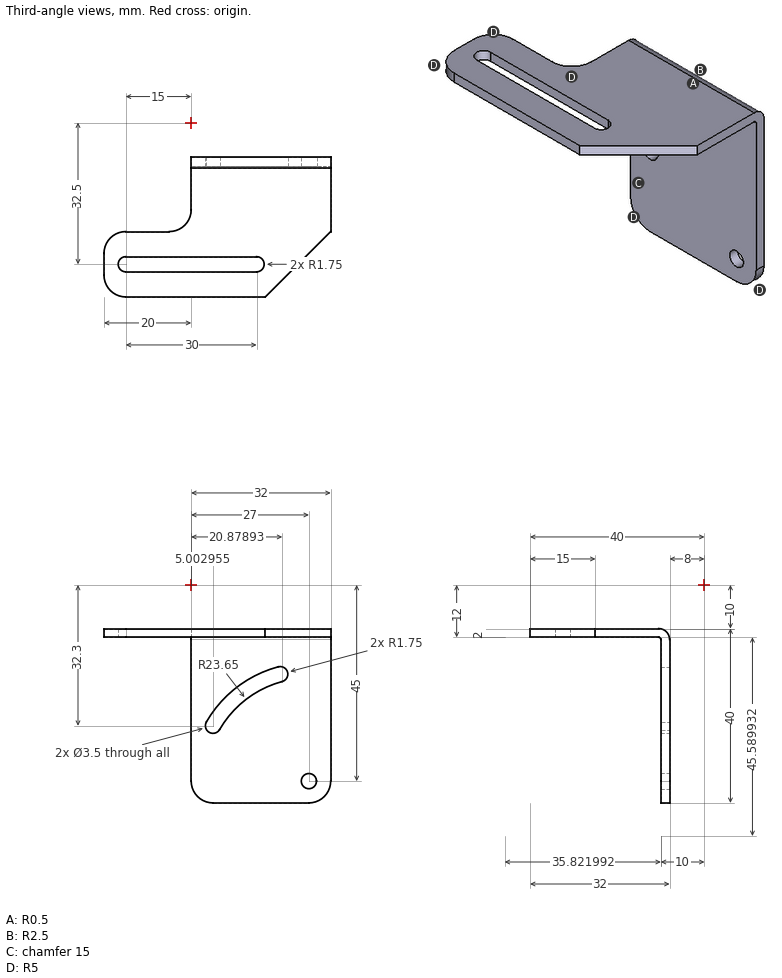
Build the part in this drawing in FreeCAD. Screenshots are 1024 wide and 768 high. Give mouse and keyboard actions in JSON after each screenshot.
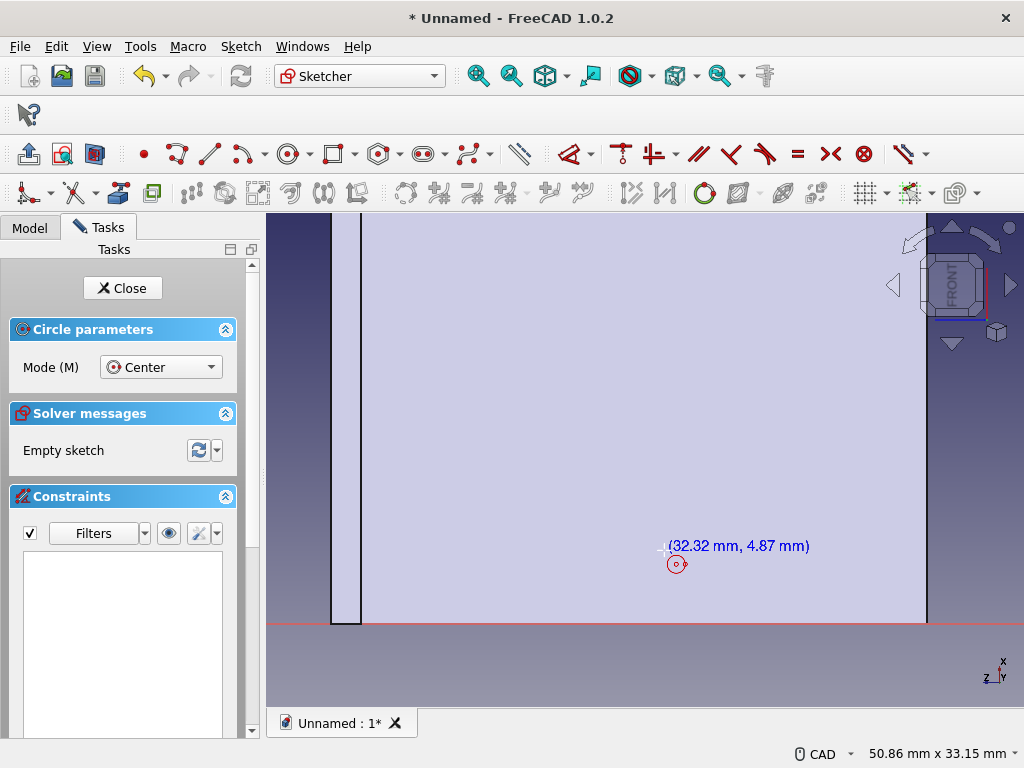
{"action": "left_click", "coordinate": [663, 549]}
{"action": "mouse_move", "coordinate": [682, 531]}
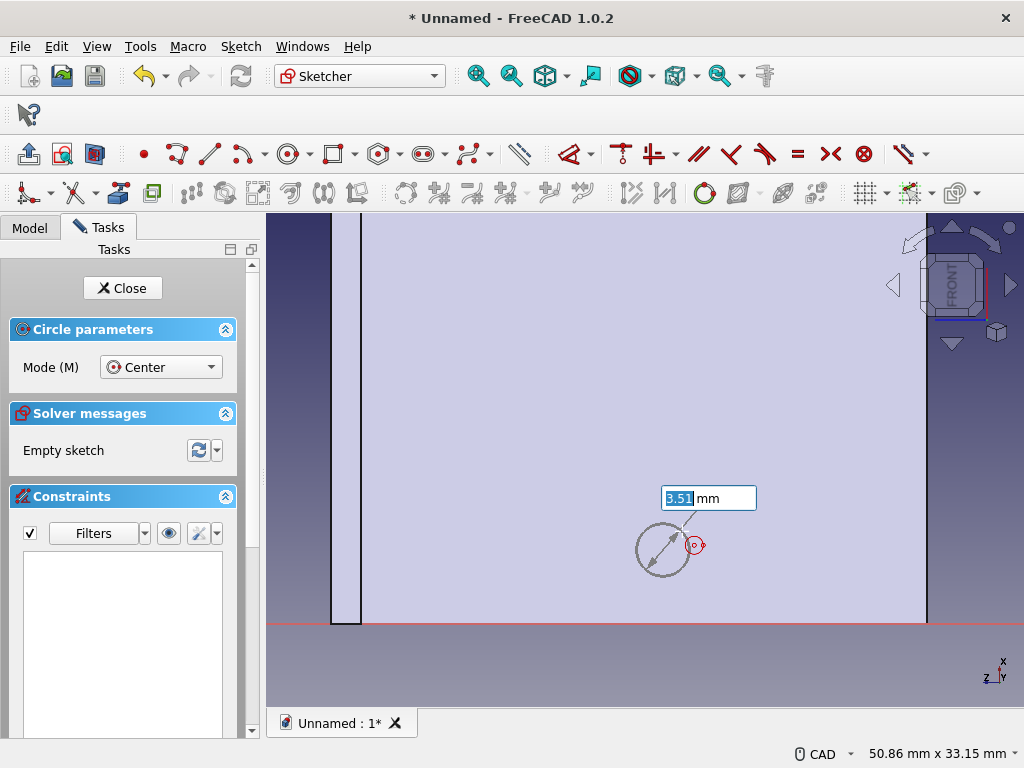
{"action": "type", "text": "3.5"}
{"action": "key", "text": "Return"}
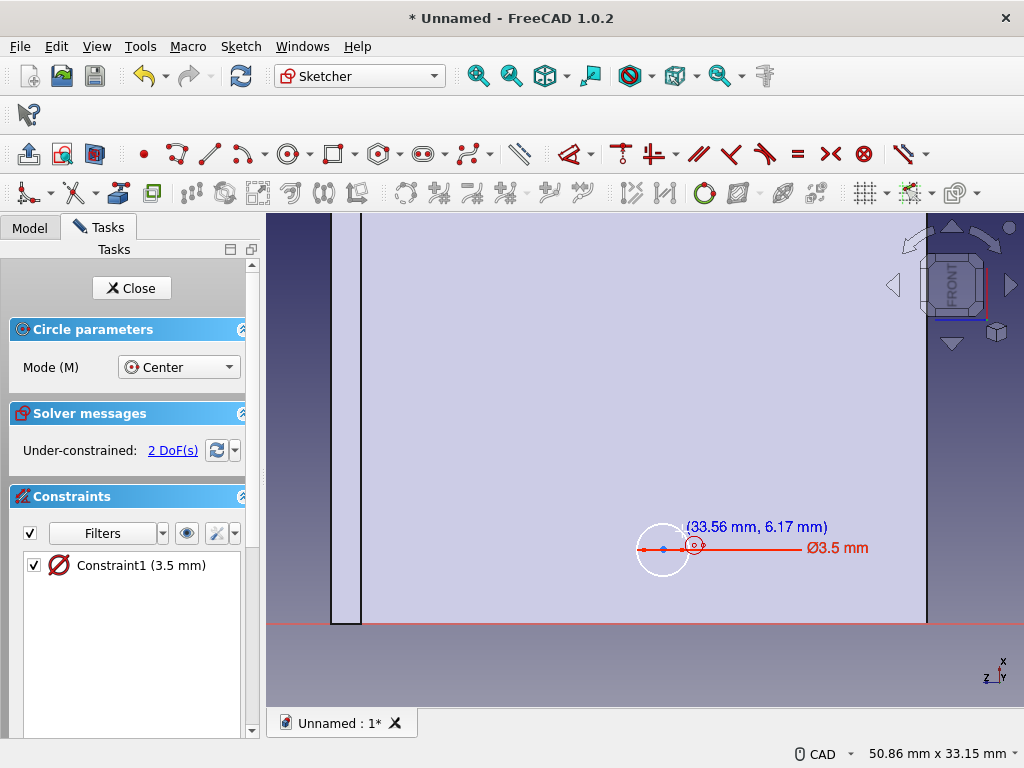
{"action": "scroll", "coordinate": [633, 521], "scroll_direction": "down", "scroll_amount": 3}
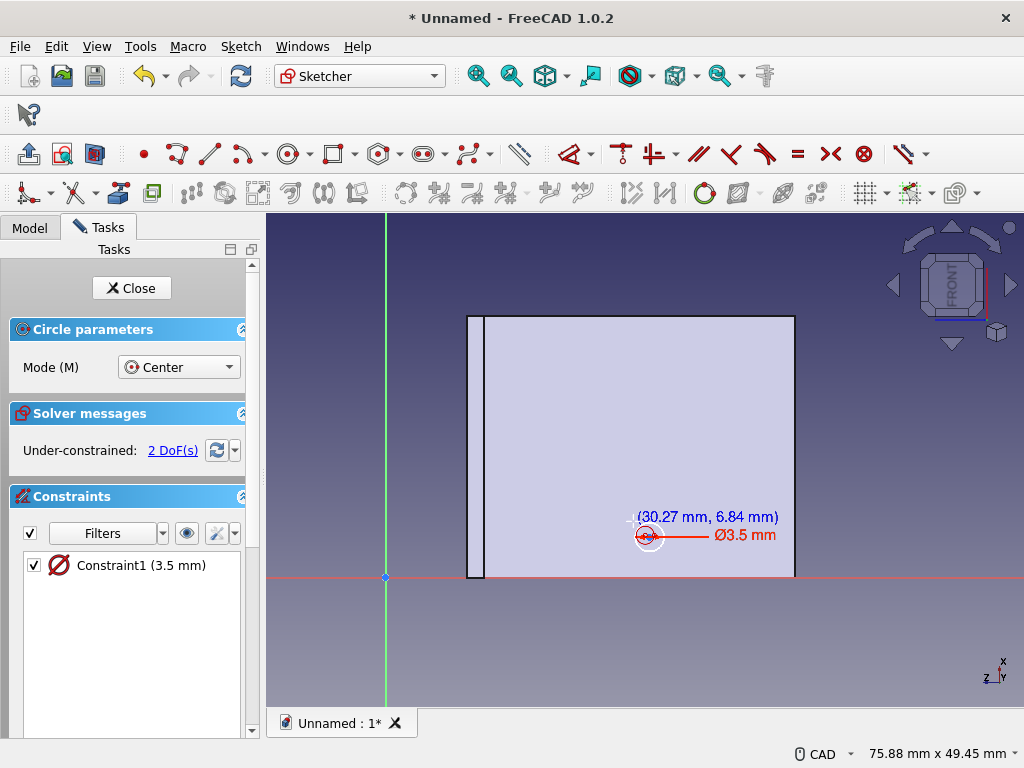
{"action": "scroll", "coordinate": [754, 357], "scroll_direction": "up", "scroll_amount": 3}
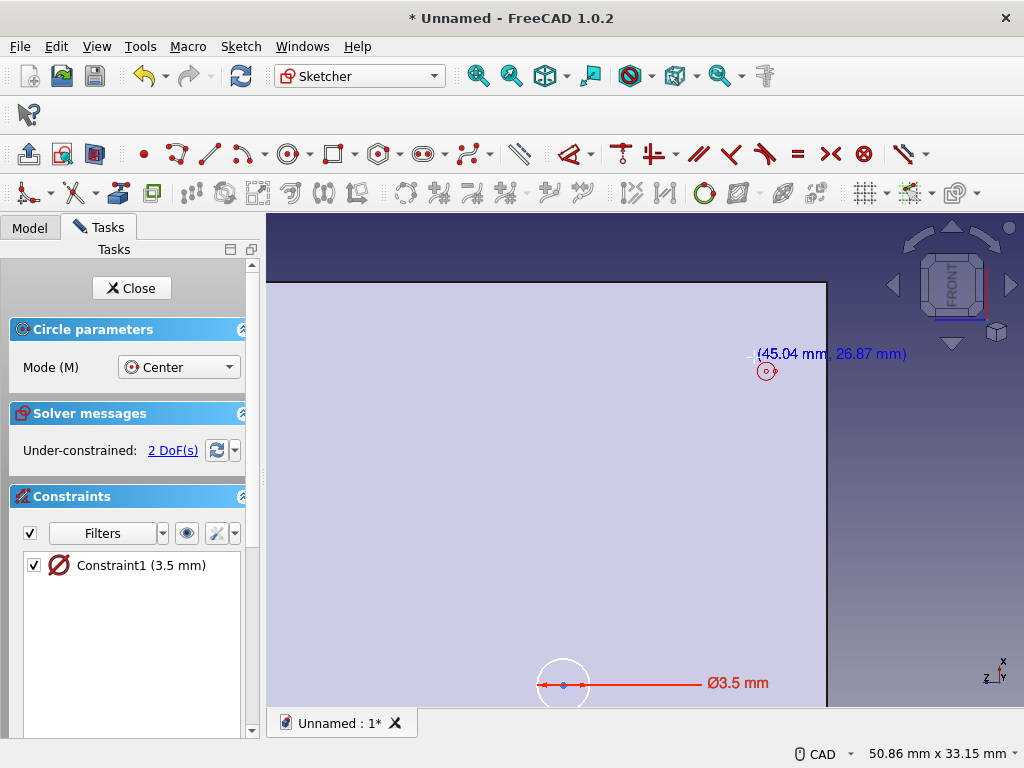
{"action": "left_click", "coordinate": [753, 357]}
{"action": "mouse_move", "coordinate": [771, 338]}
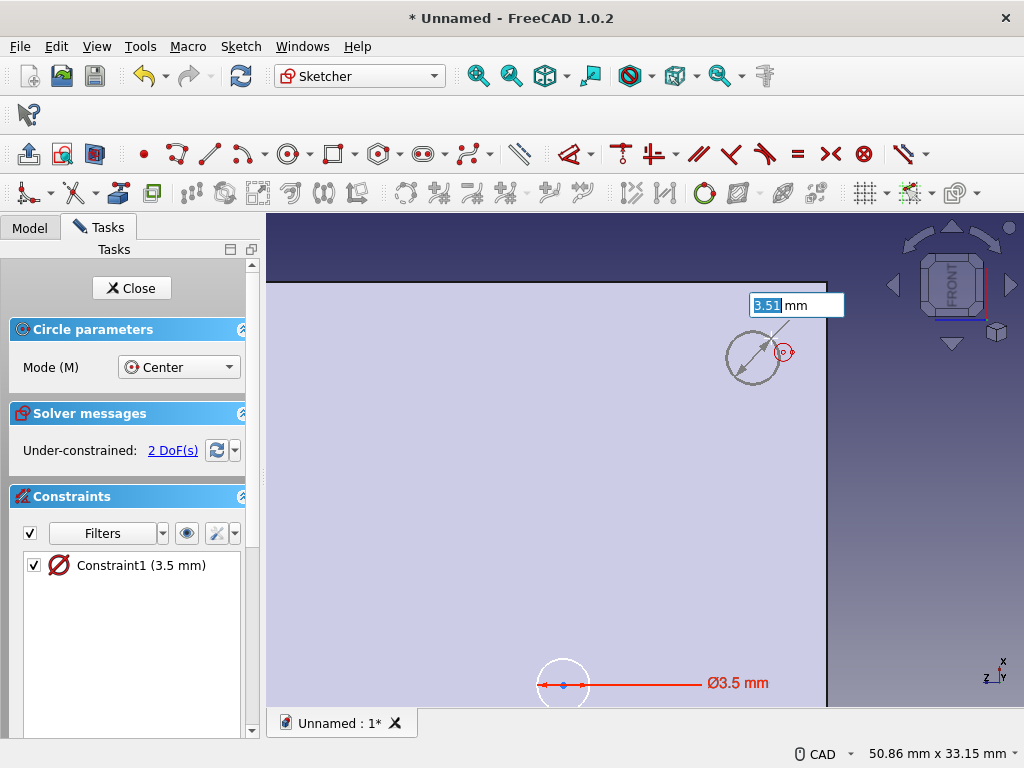
{"action": "type", "text": "3.5"}
{"action": "key", "text": "Return"}
{"action": "key", "text": "Escape"}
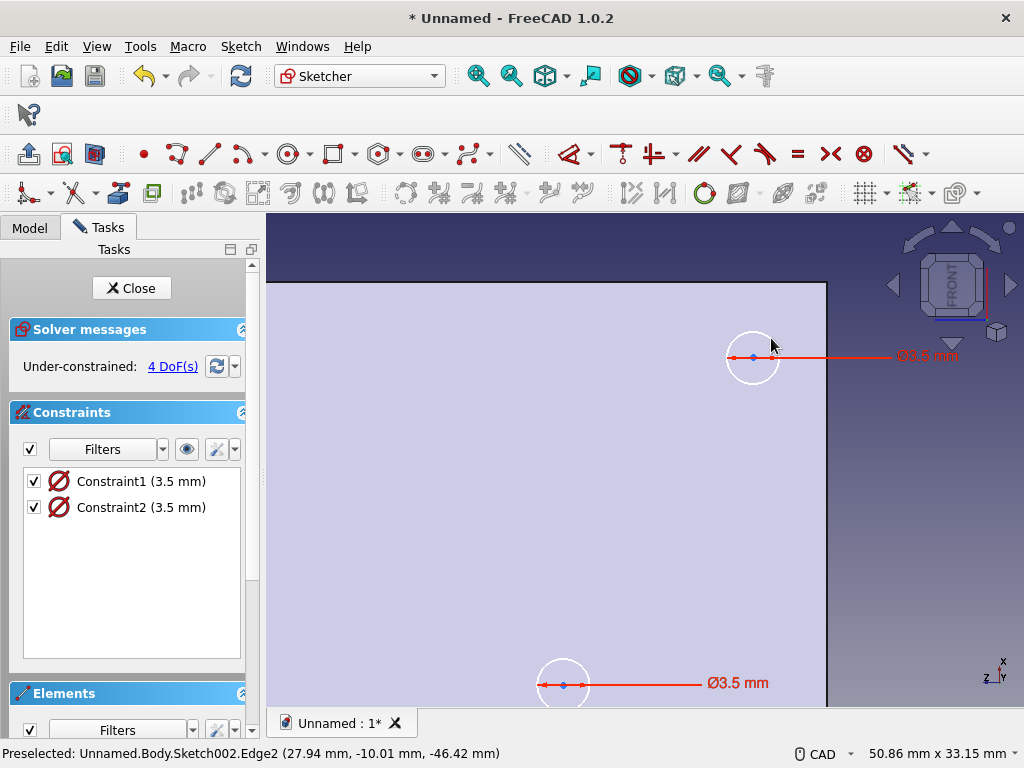
{"action": "key", "text": "d"}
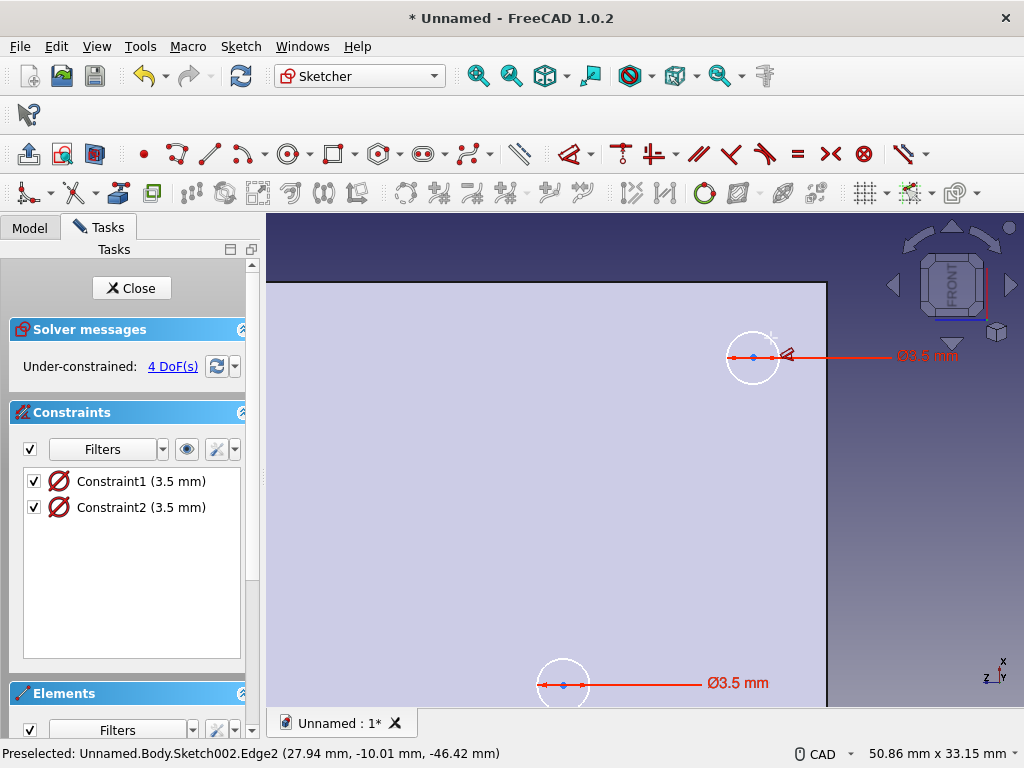
{"action": "left_click", "coordinate": [753, 358]}
{"action": "left_click", "coordinate": [523, 324]}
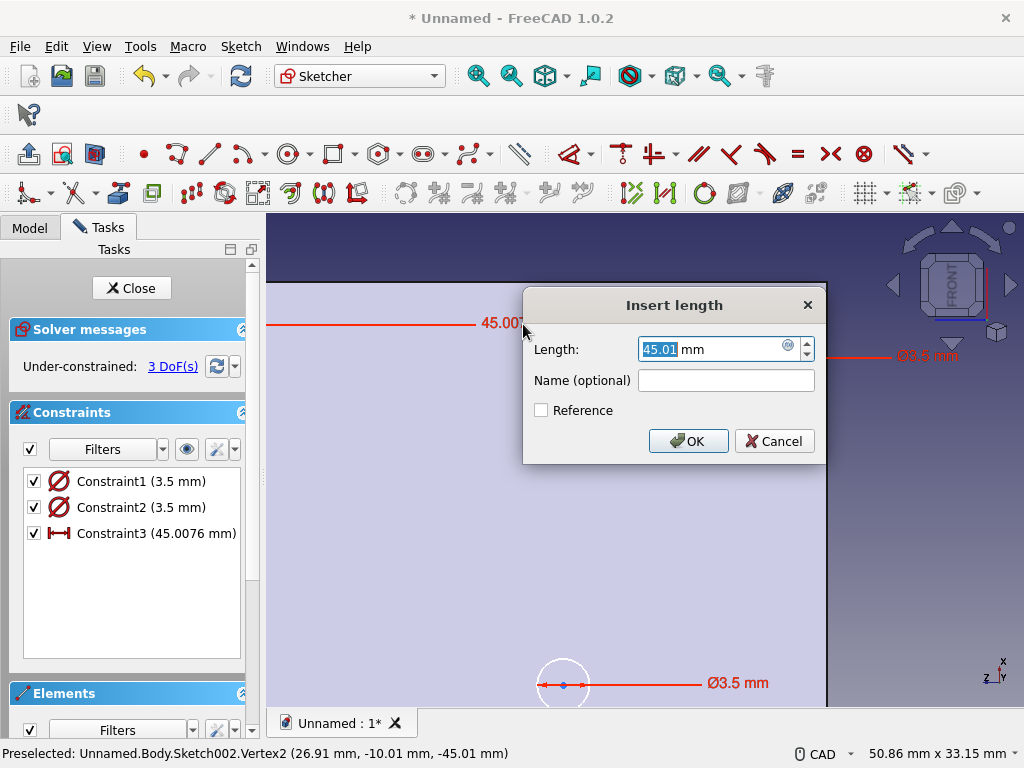
{"action": "type", "text": "45"}
{"action": "key", "text": "Return"}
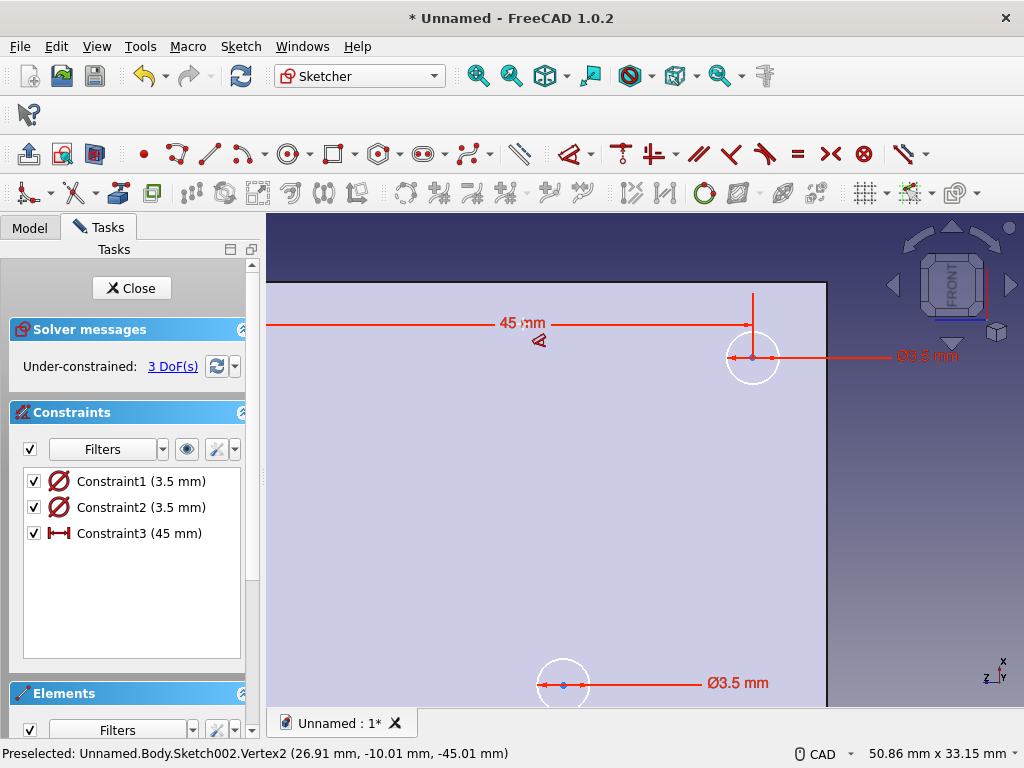
{"action": "left_click", "coordinate": [753, 358]}
{"action": "left_click", "coordinate": [787, 518]}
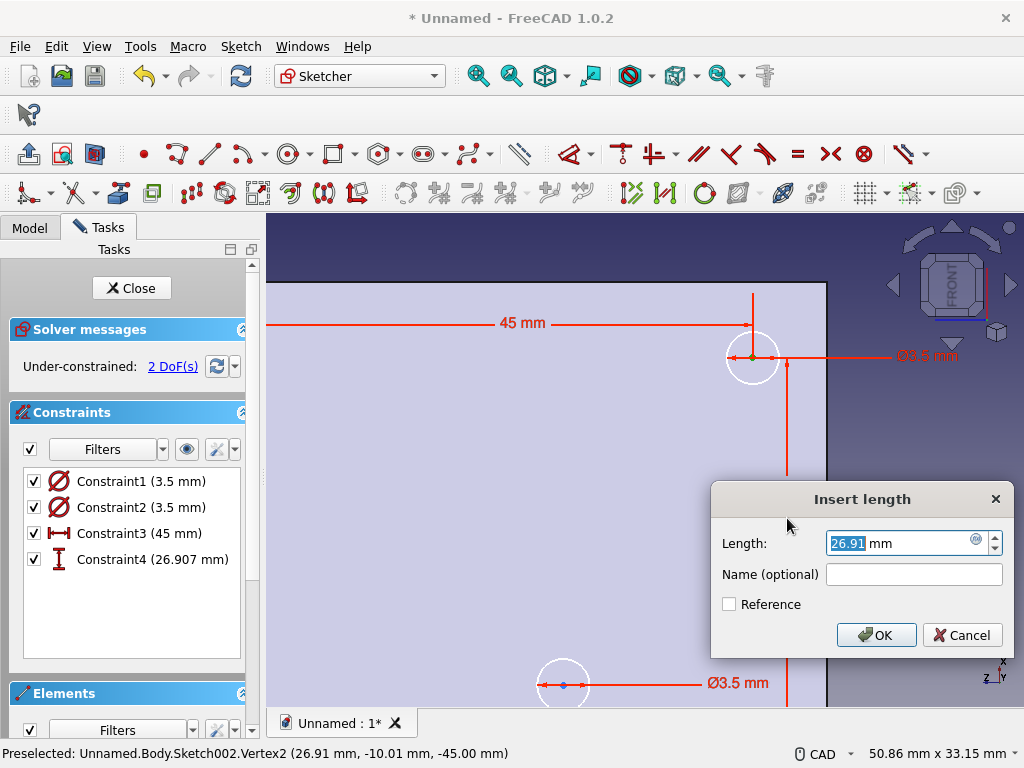
{"action": "type", "text": "27"}
{"action": "key", "text": "Return"}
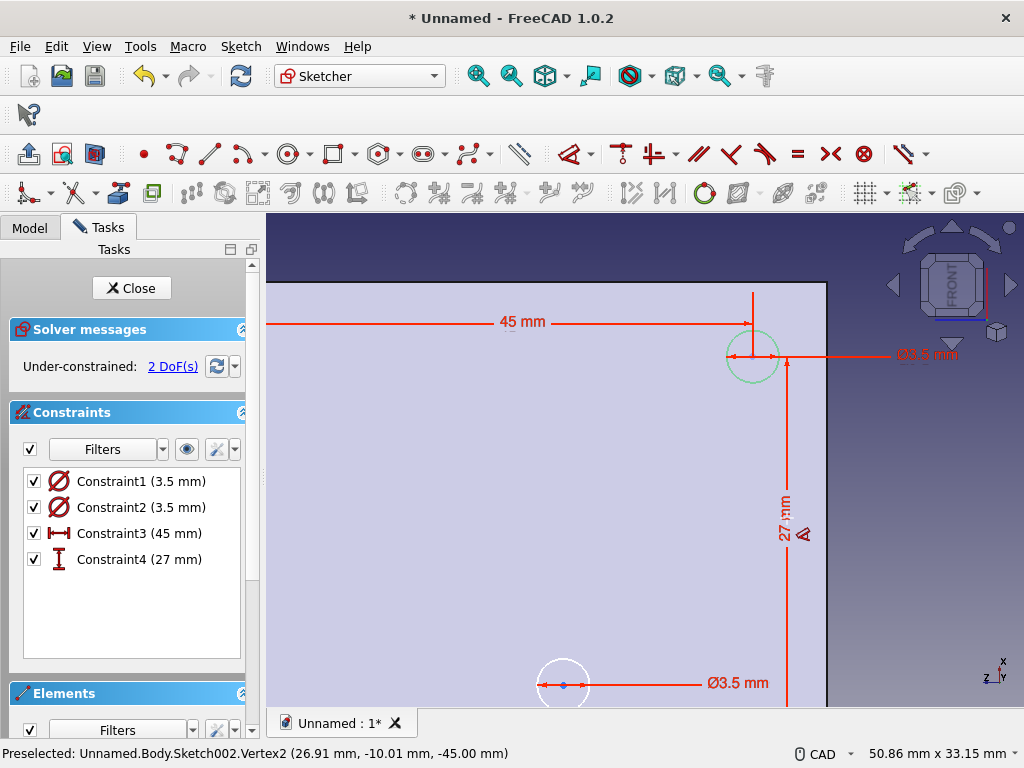
{"action": "scroll", "coordinate": [754, 357], "scroll_direction": "down", "scroll_amount": 3}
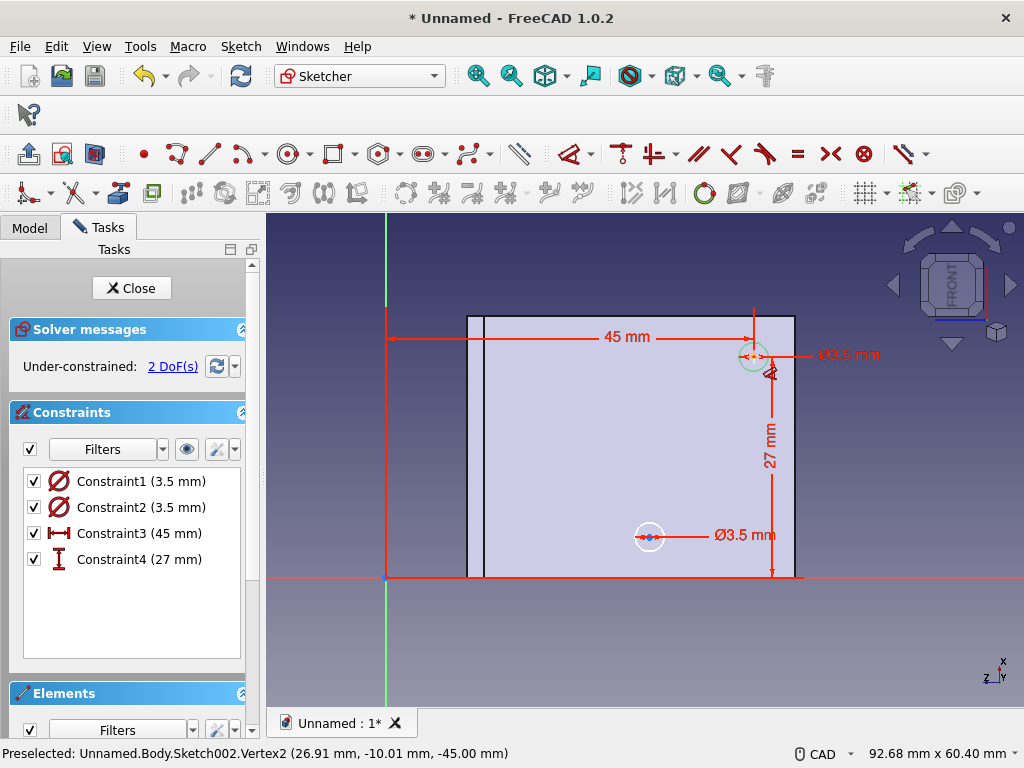
{"action": "left_click", "coordinate": [650, 537]}
{"action": "left_click", "coordinate": [518, 612]}